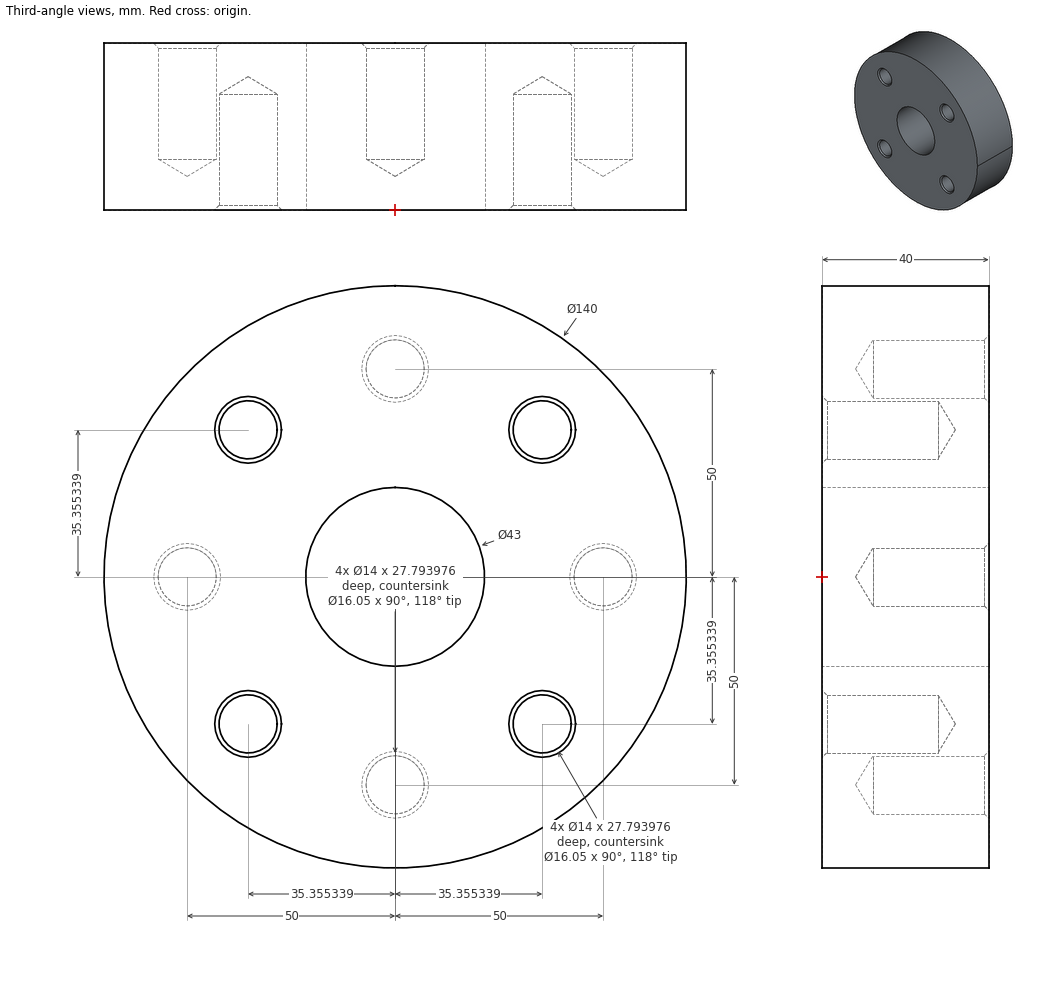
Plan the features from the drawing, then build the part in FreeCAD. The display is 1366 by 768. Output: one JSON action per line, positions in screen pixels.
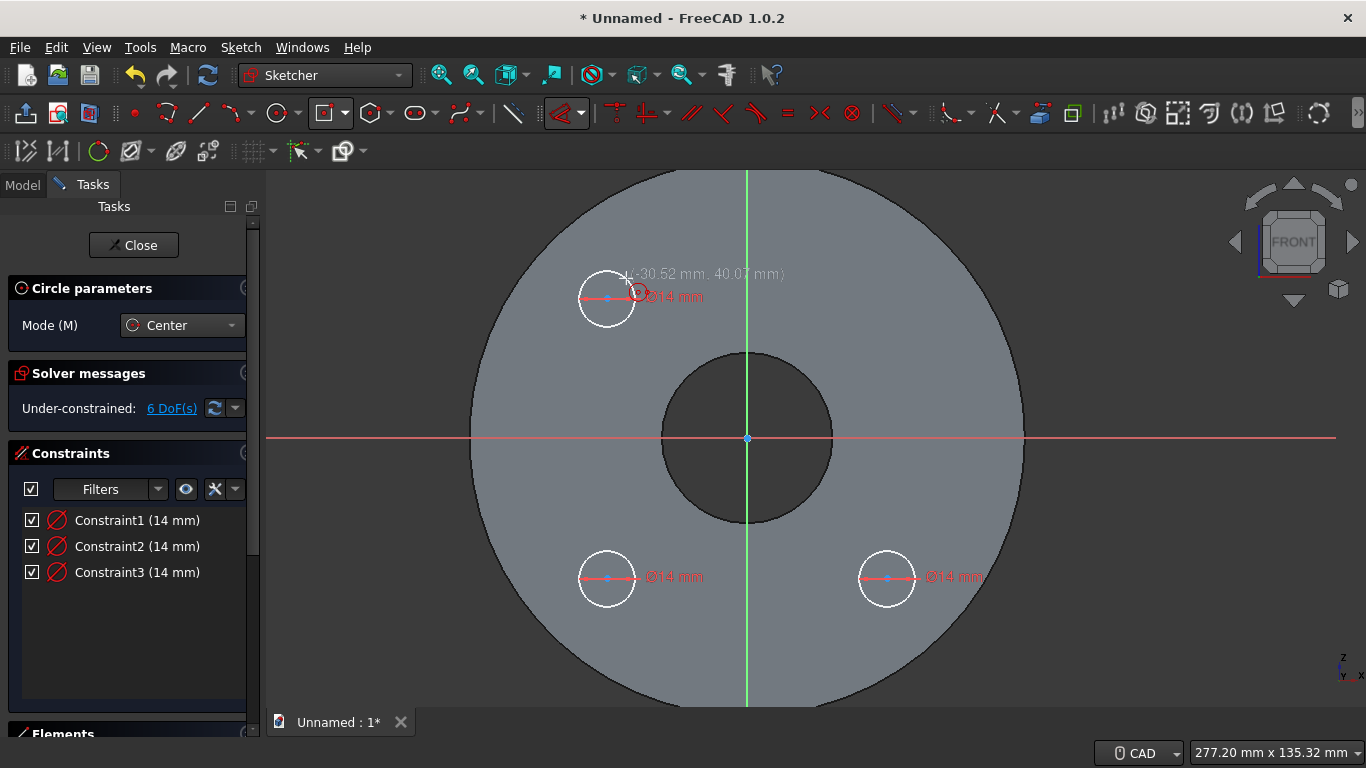
{"action": "left_click", "coordinate": [887, 298]}
{"action": "mouse_move", "coordinate": [907, 278]}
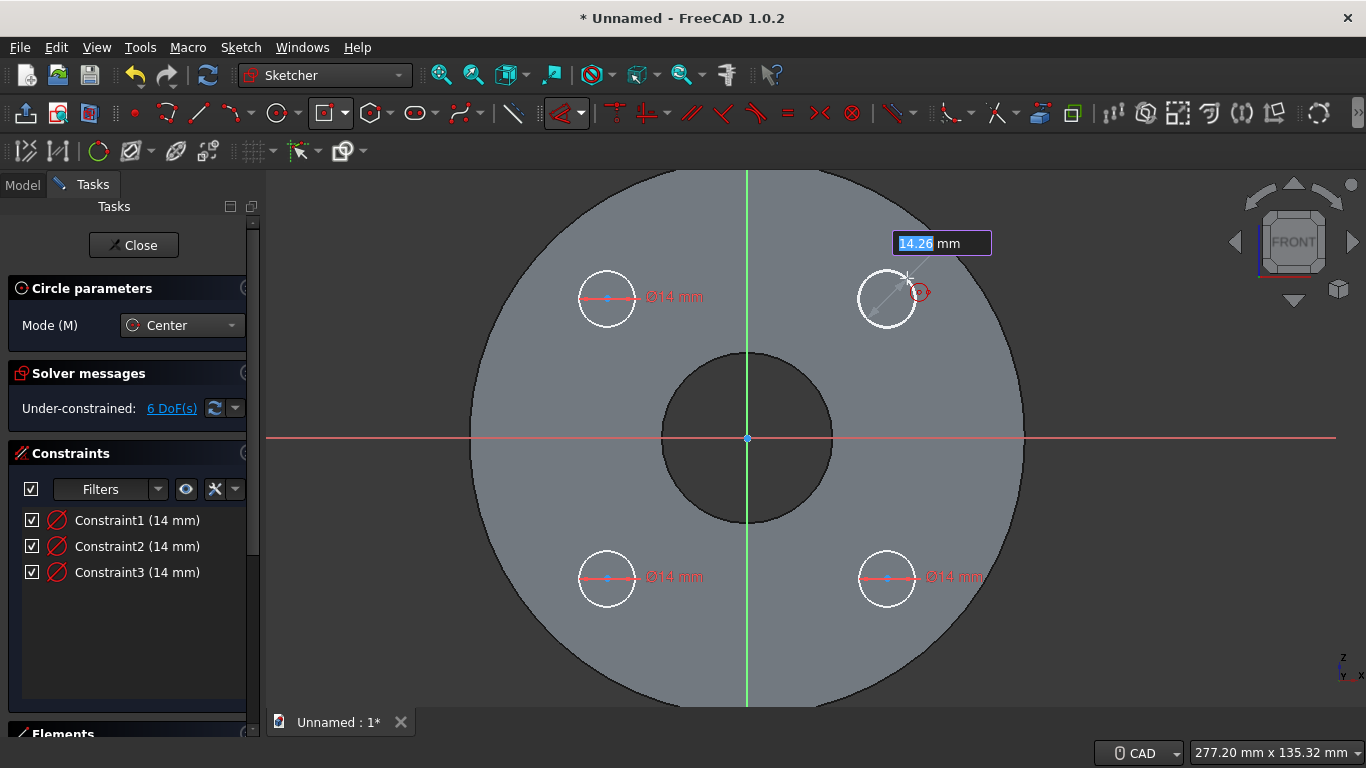
{"action": "type", "text": "14"}
{"action": "key", "text": "Return"}
{"action": "key", "text": "Escape"}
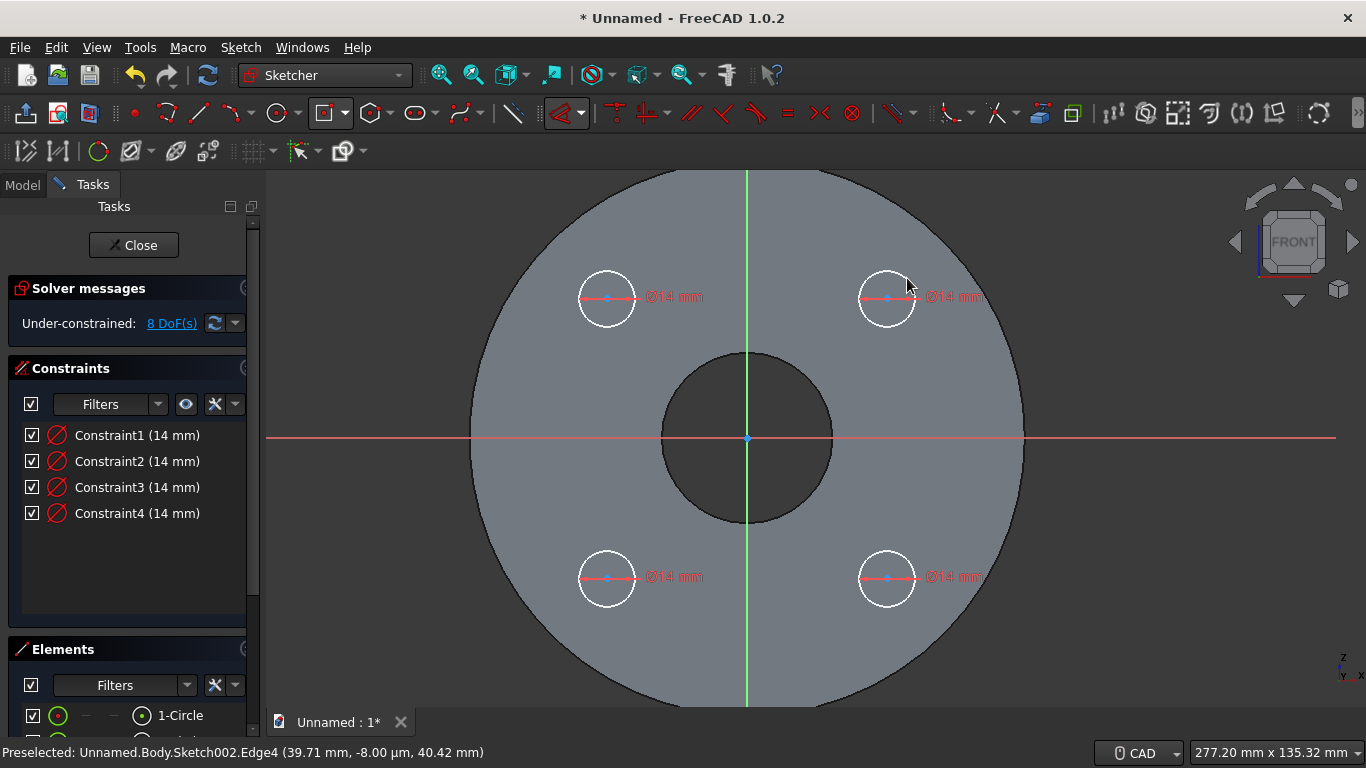
{"action": "left_click", "coordinate": [887, 579]}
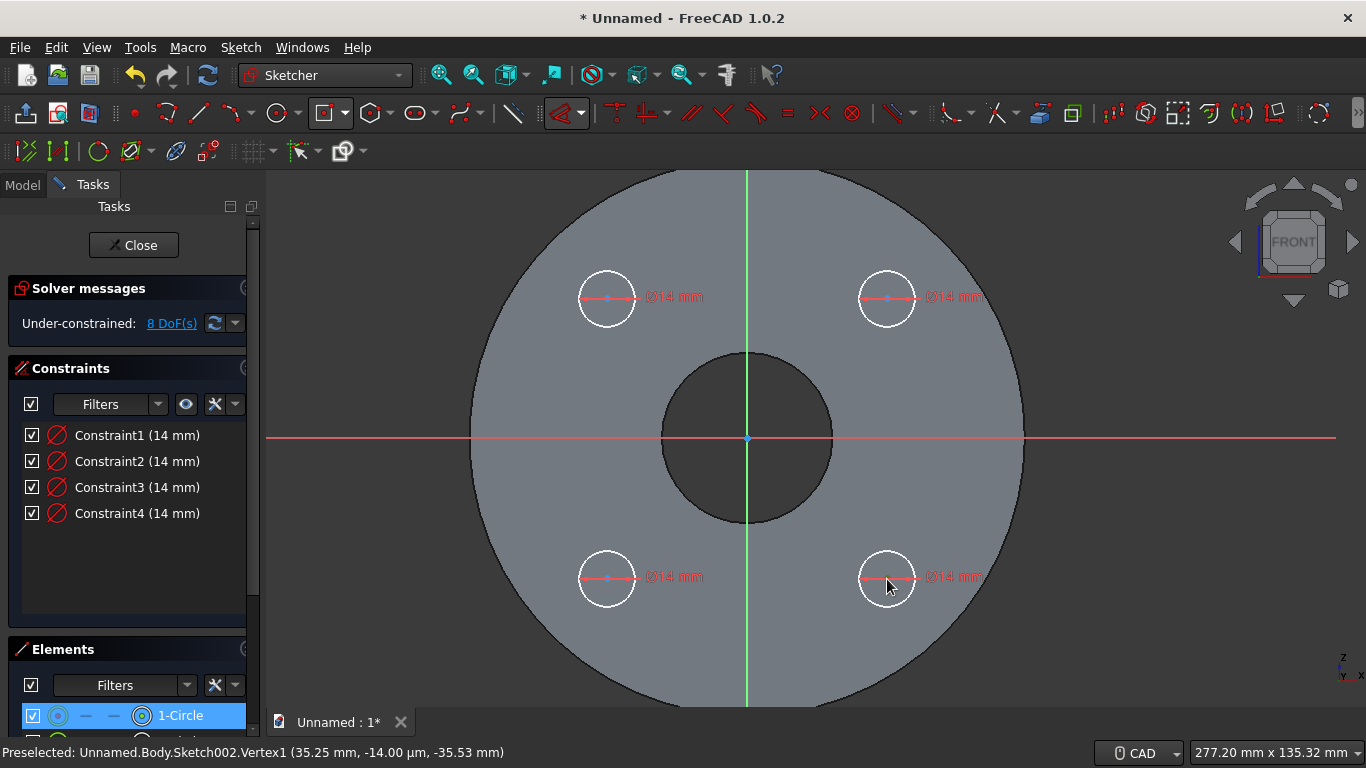
{"action": "left_click", "coordinate": [607, 579]}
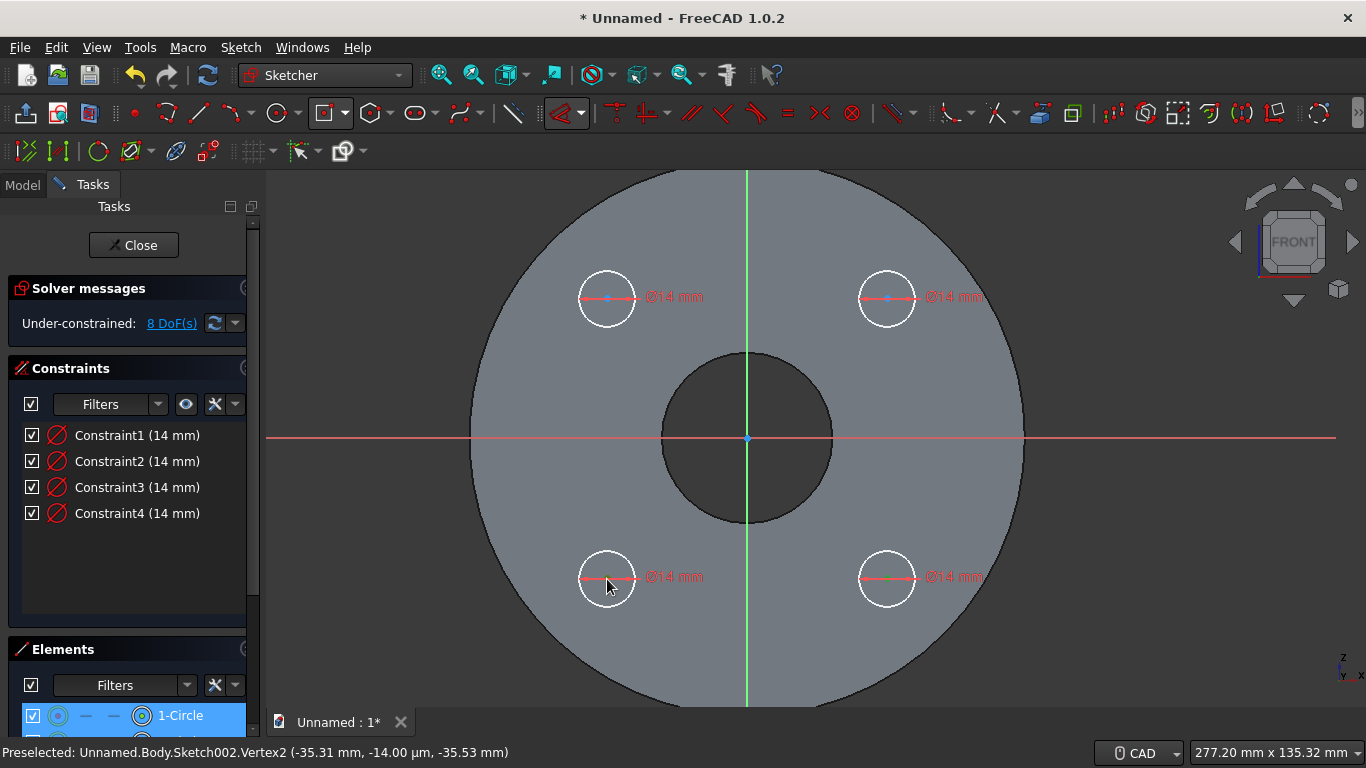
{"action": "left_click", "coordinate": [670, 114]}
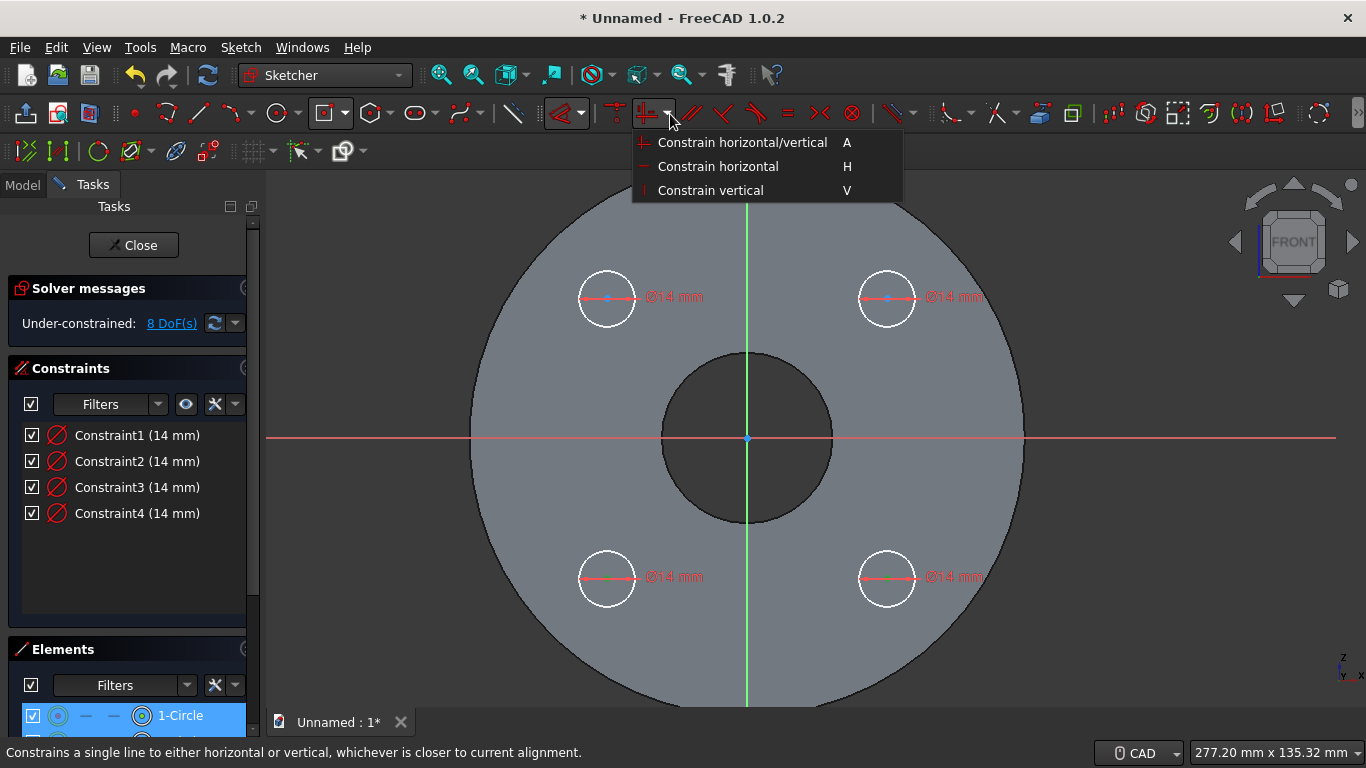
{"action": "left_click", "coordinate": [768, 166]}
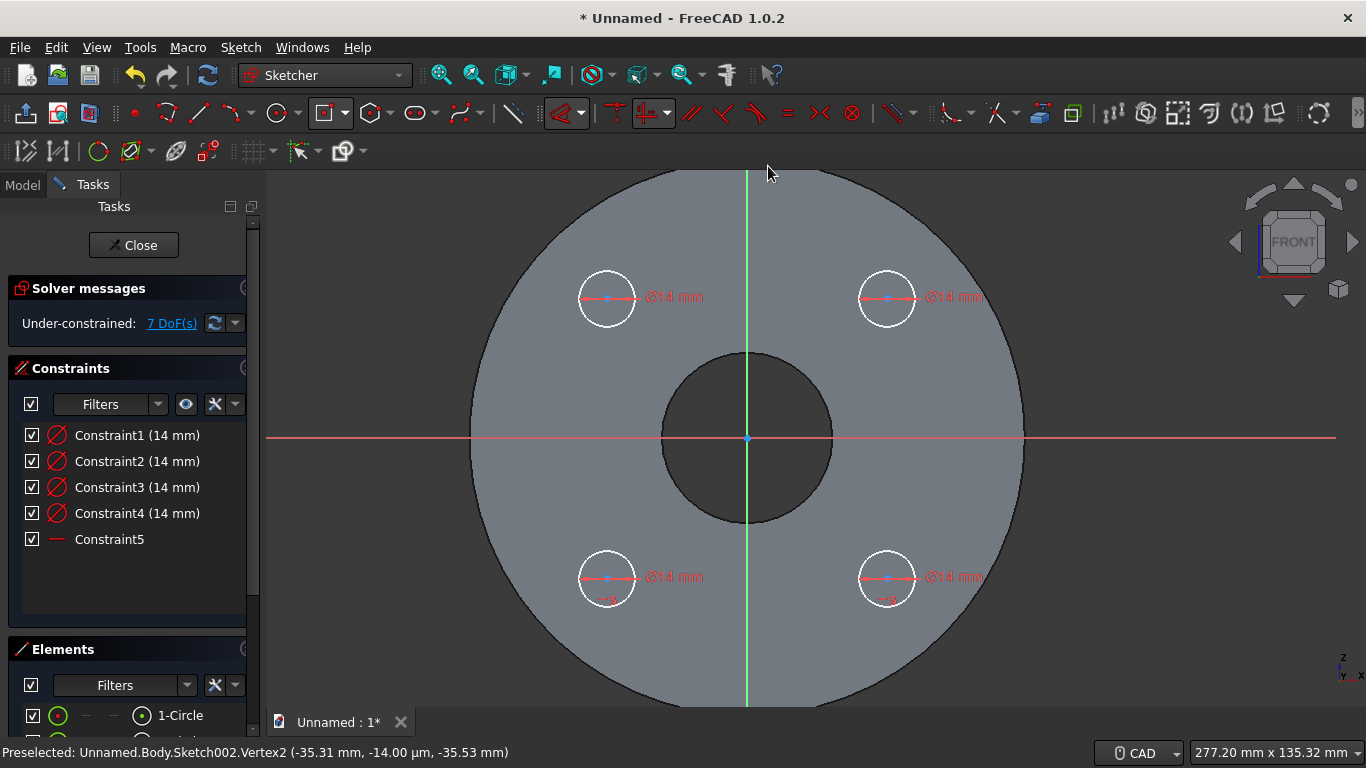
{"action": "left_click", "coordinate": [607, 579]}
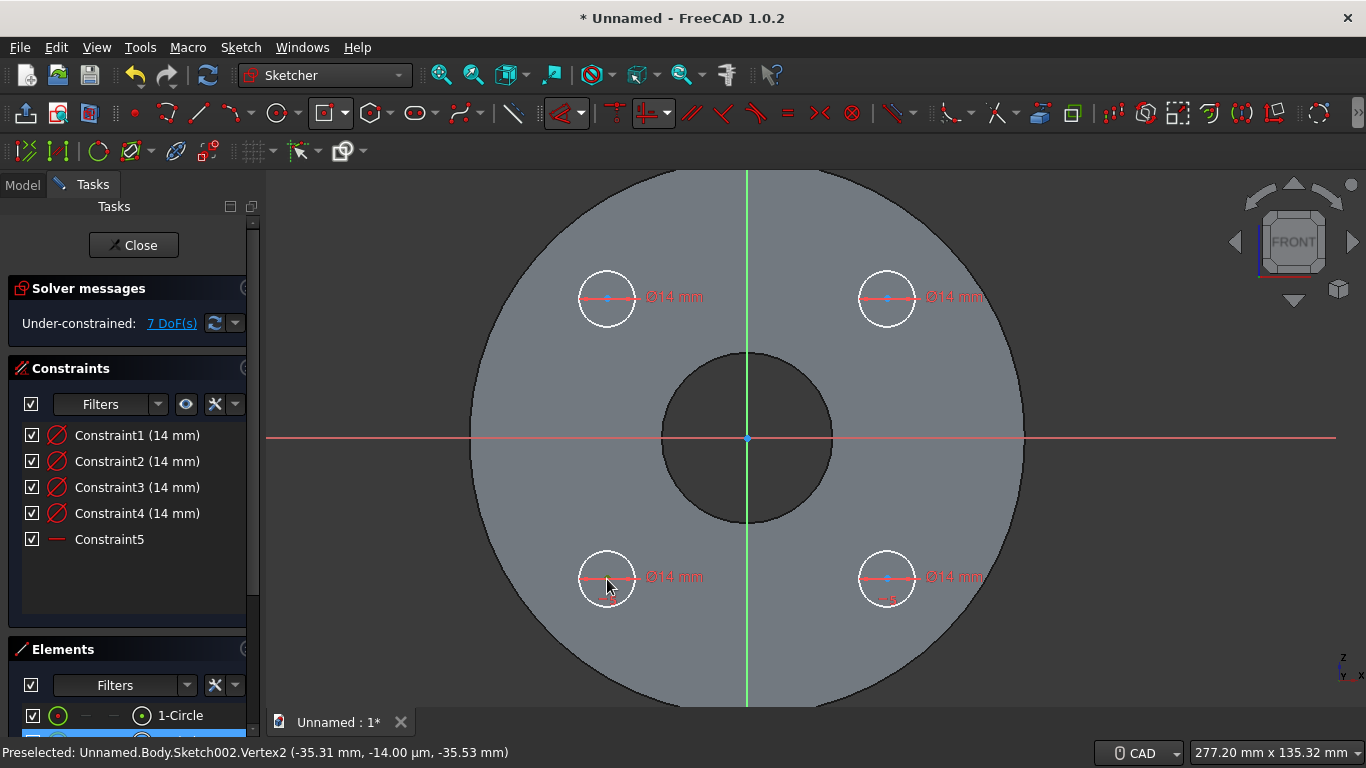
{"action": "left_click", "coordinate": [607, 299]}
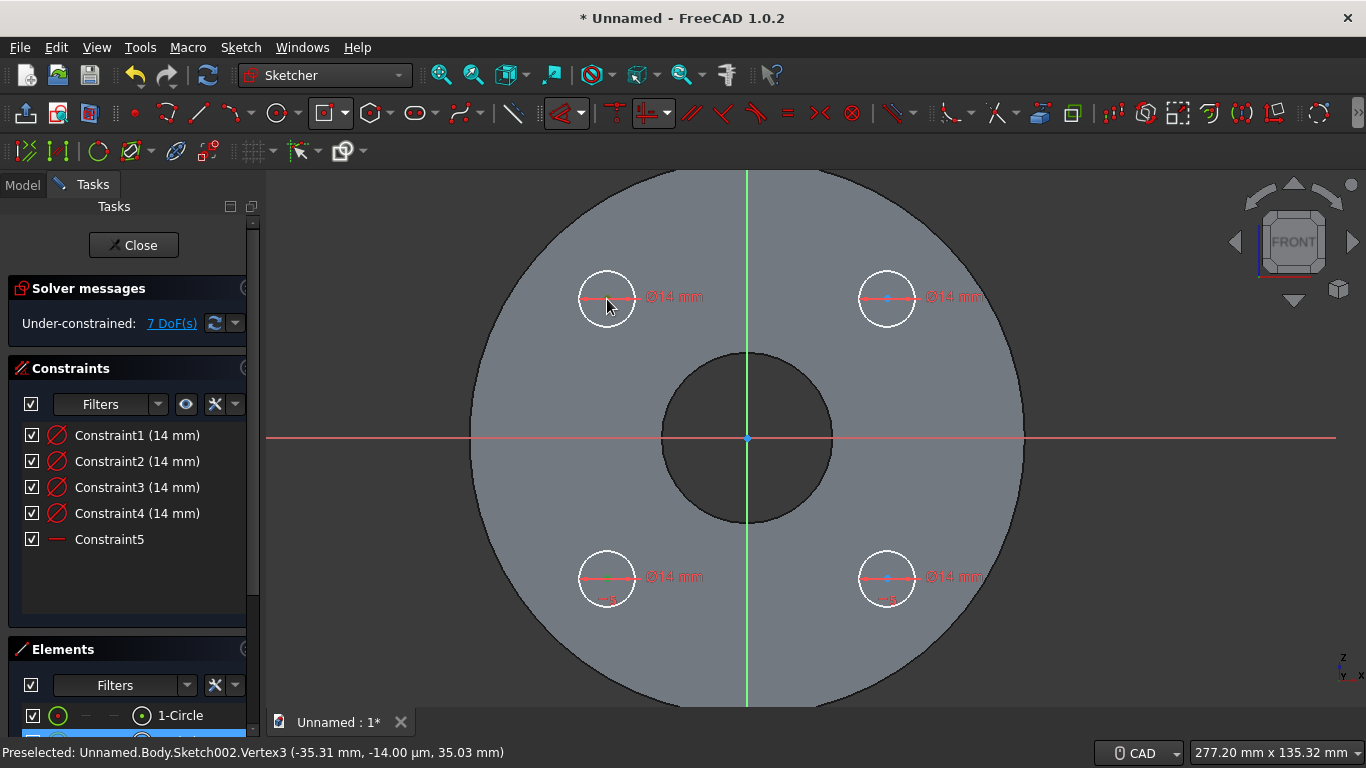
{"action": "key", "text": "v"}